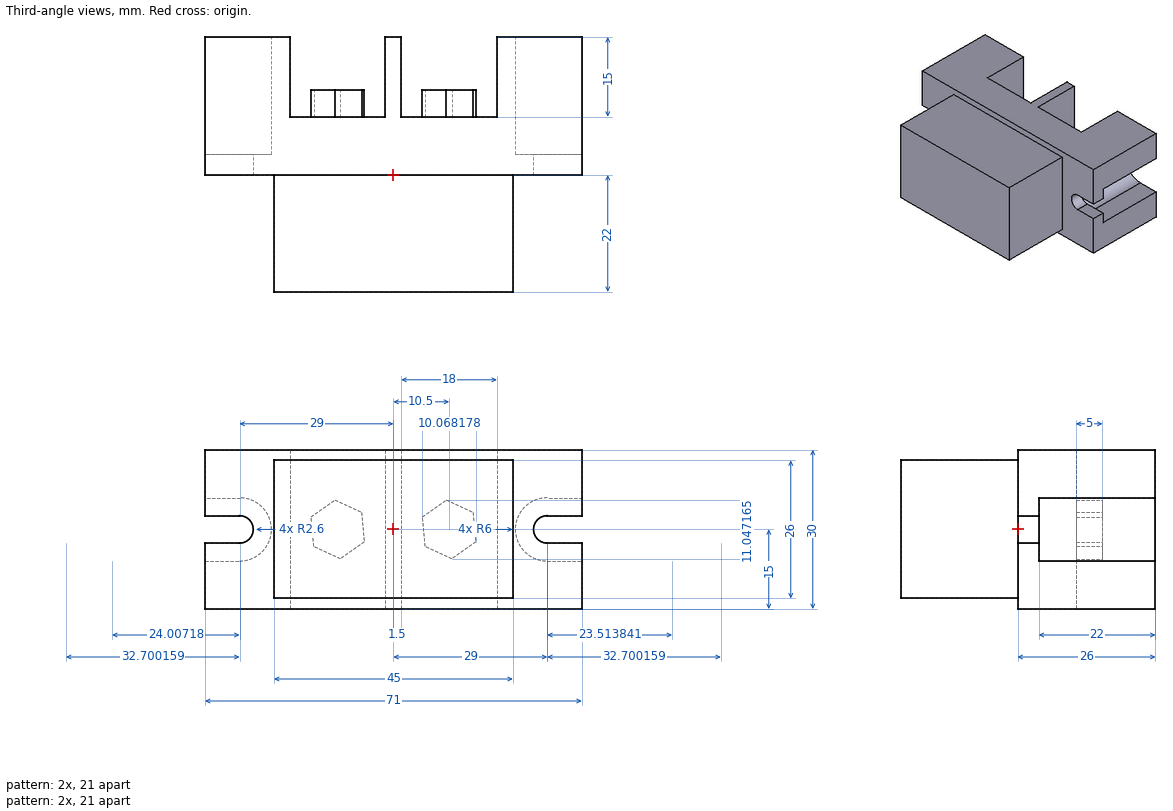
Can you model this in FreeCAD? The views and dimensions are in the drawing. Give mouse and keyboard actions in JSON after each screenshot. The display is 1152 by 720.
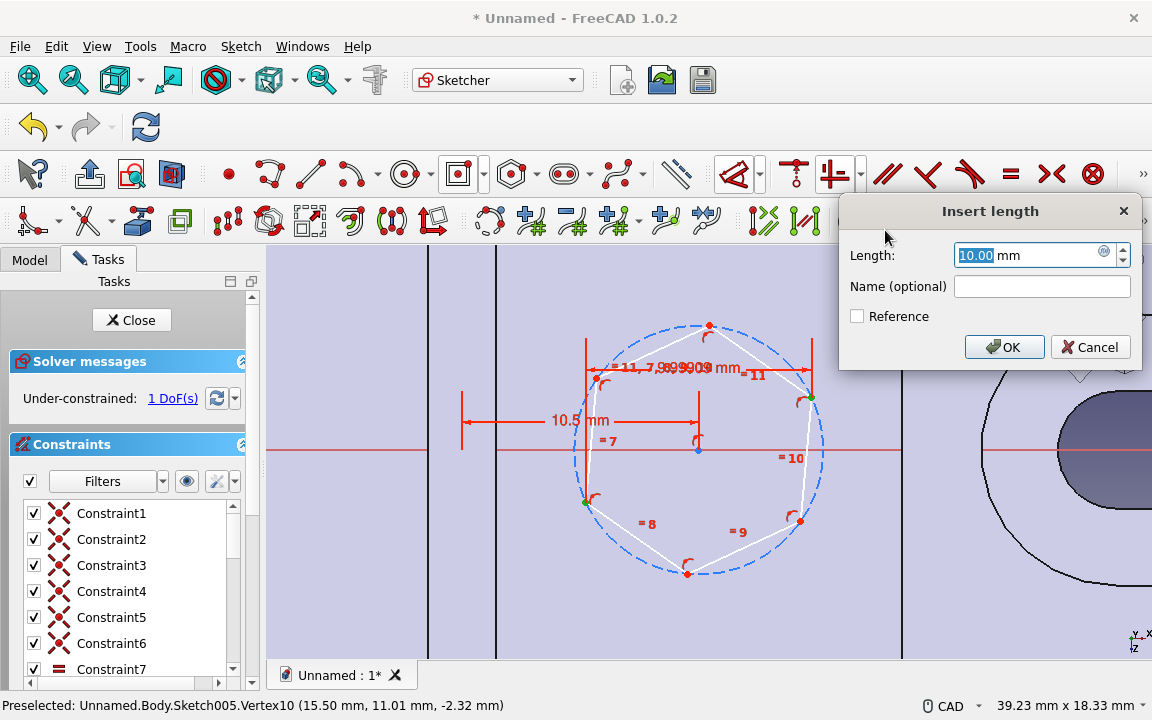
{"action": "type", "text": "10.068178"}
{"action": "key", "text": "Return"}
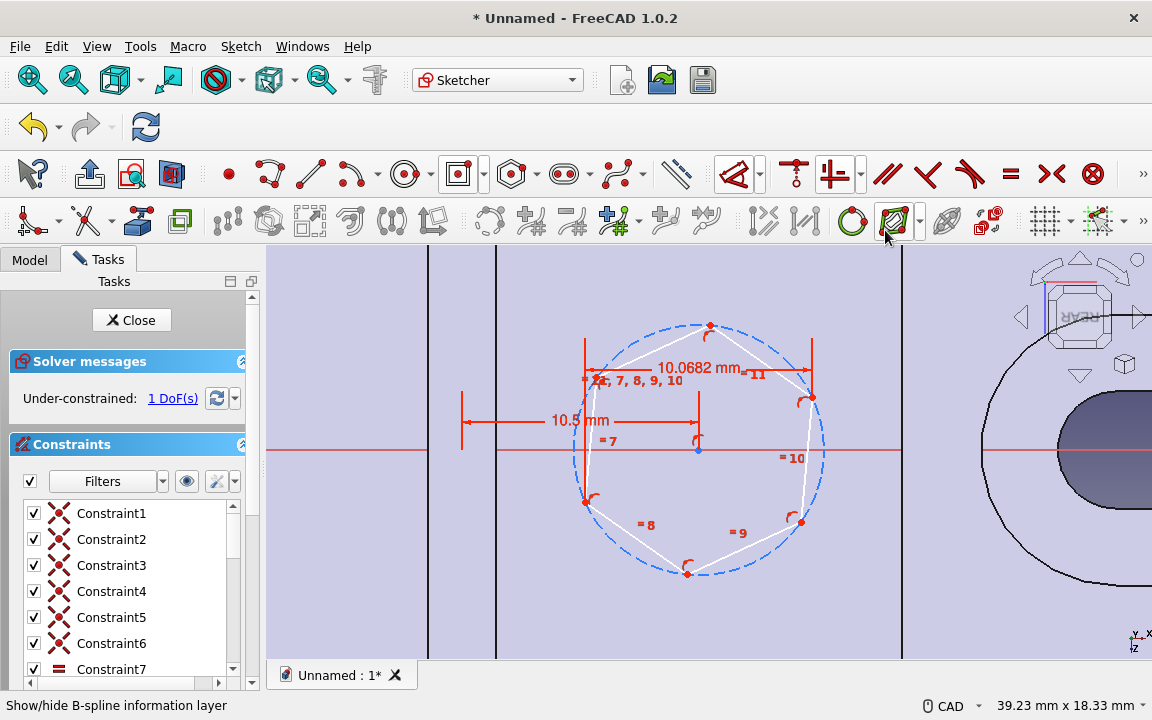
{"action": "left_click", "coordinate": [687, 575]}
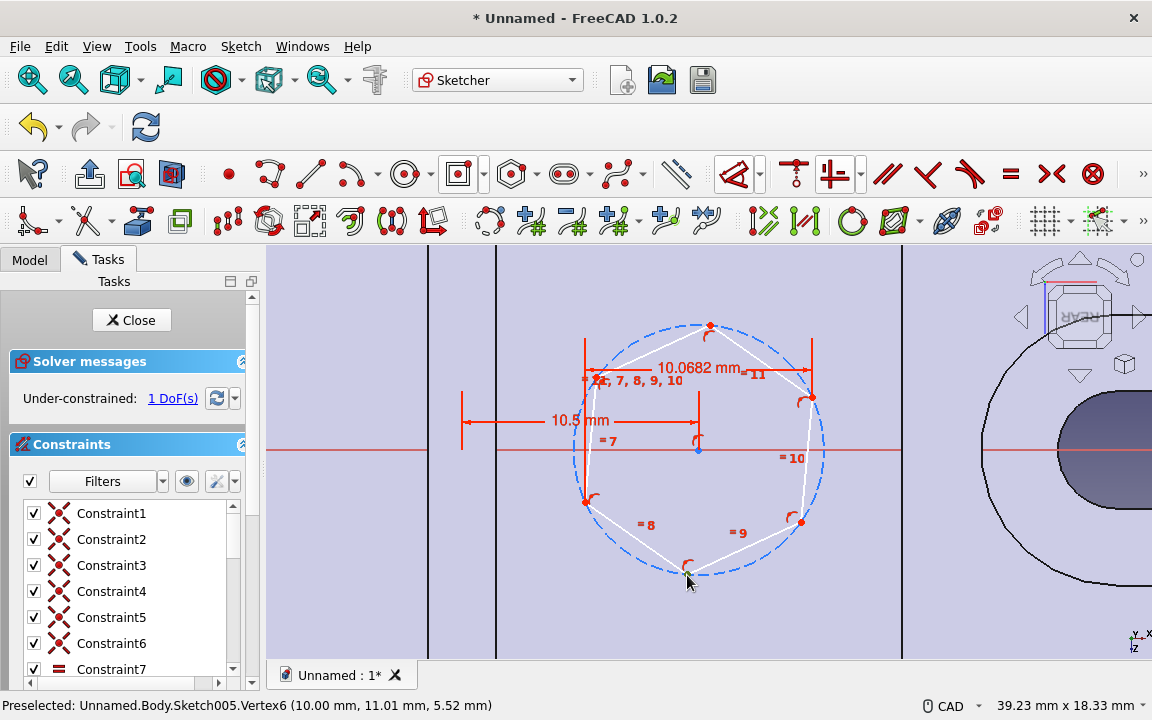
{"action": "left_click", "coordinate": [710, 325]}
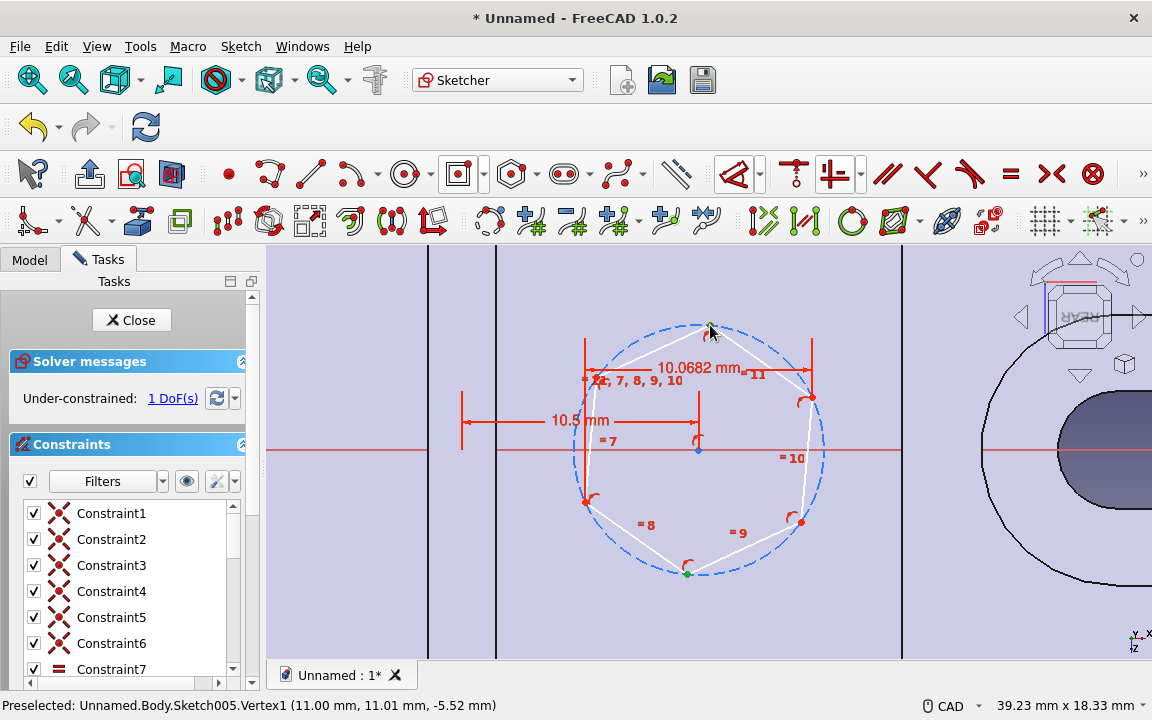
{"action": "key", "text": "i"}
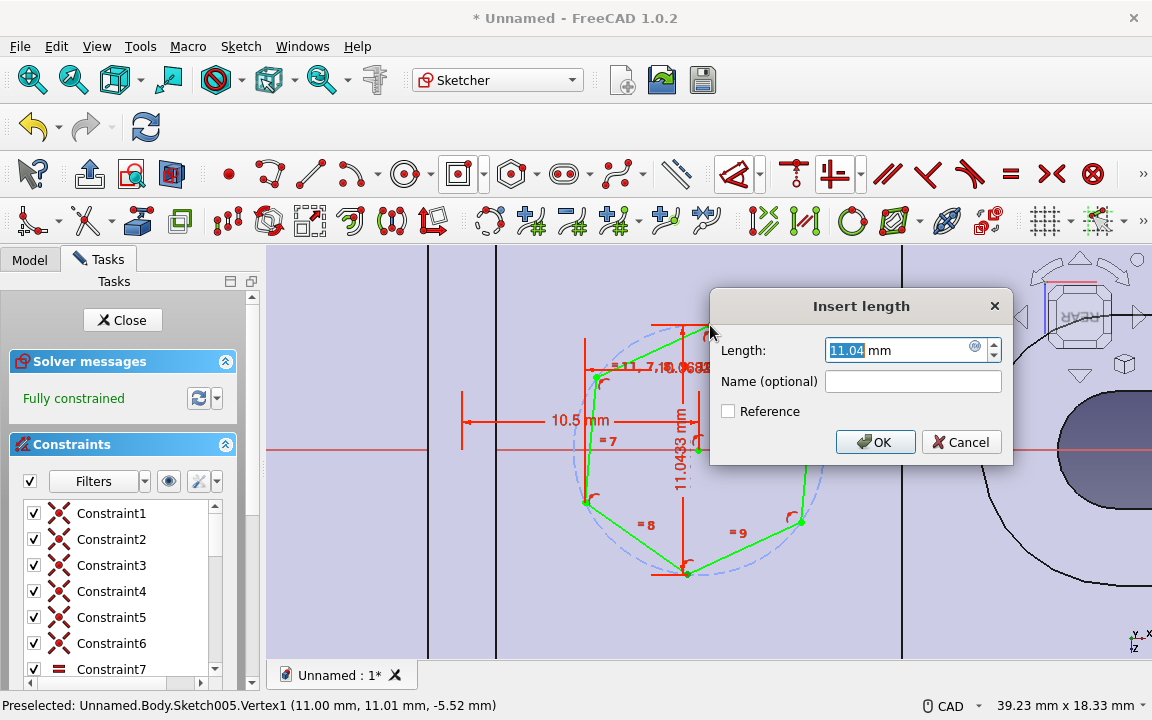
{"action": "type", "text": "11.047165"}
{"action": "key", "text": "Return"}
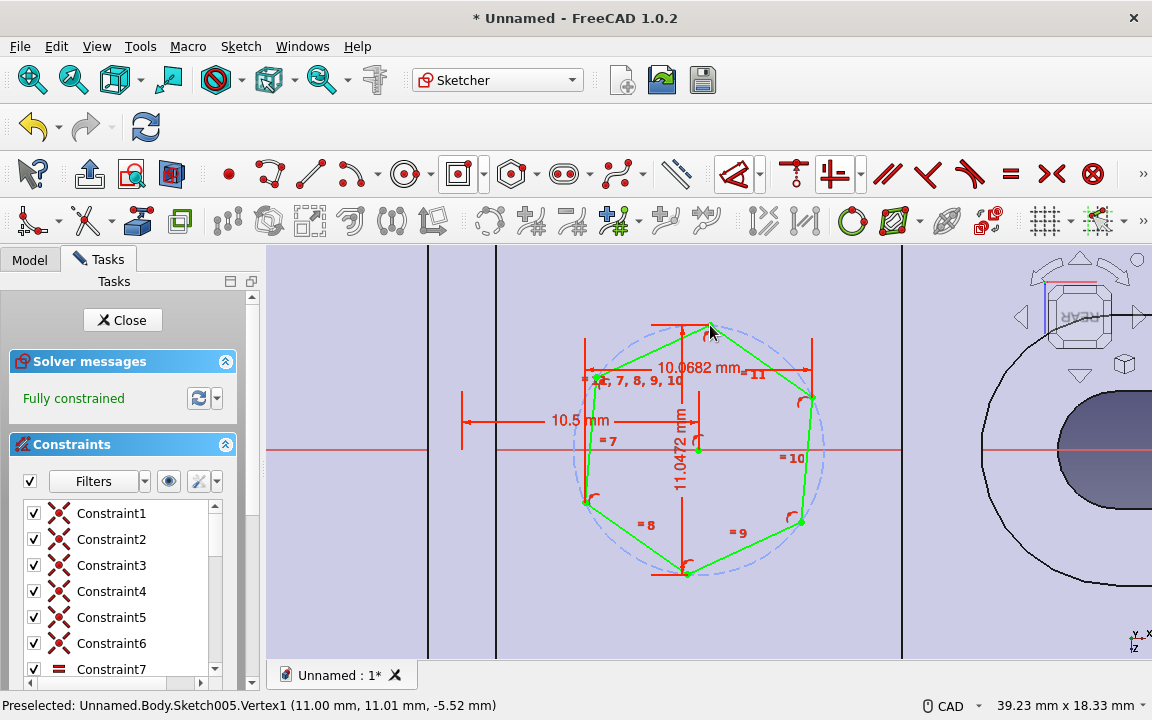
{"action": "left_click", "coordinate": [123, 320]}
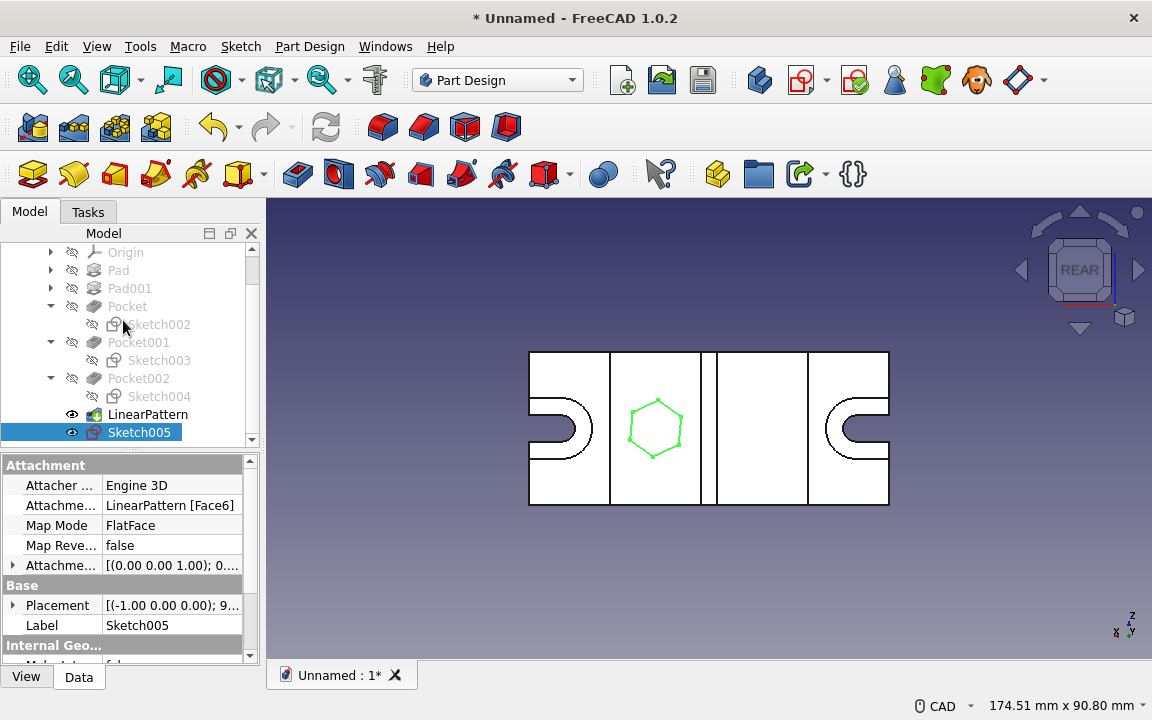
{"action": "left_click", "coordinate": [33, 174]}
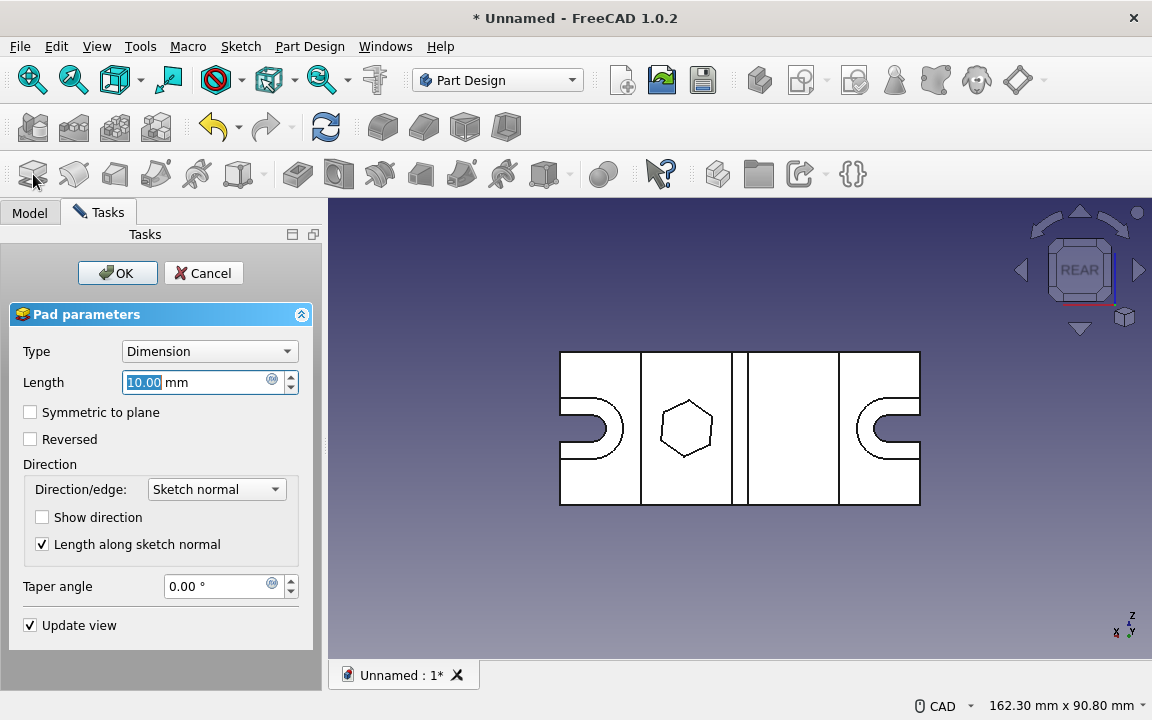
{"action": "type", "text": "5"}
{"action": "key", "text": "Tab"}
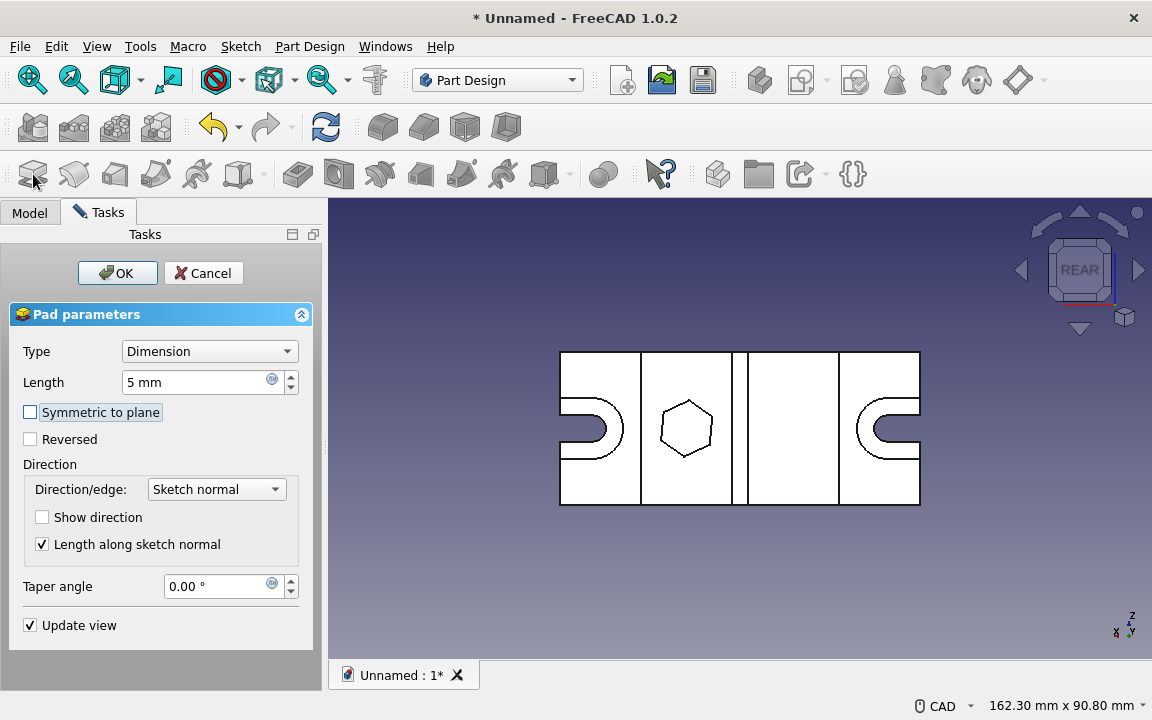
{"action": "left_click", "coordinate": [118, 273]}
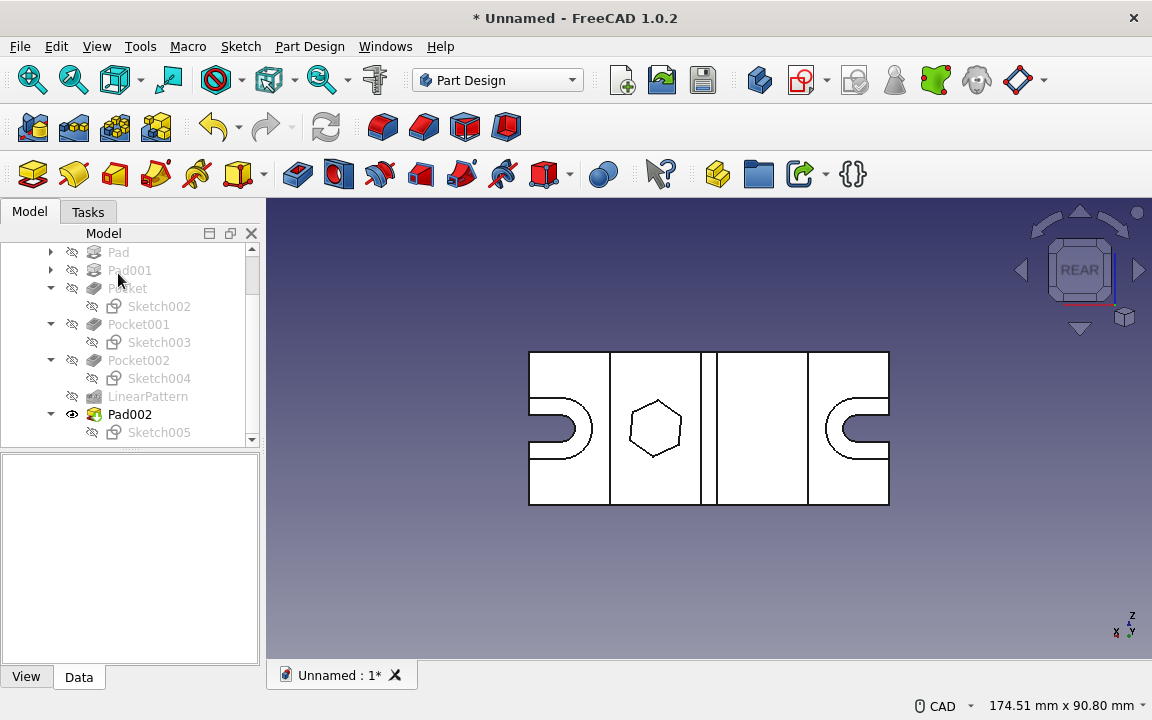
{"action": "key", "text": "v f"}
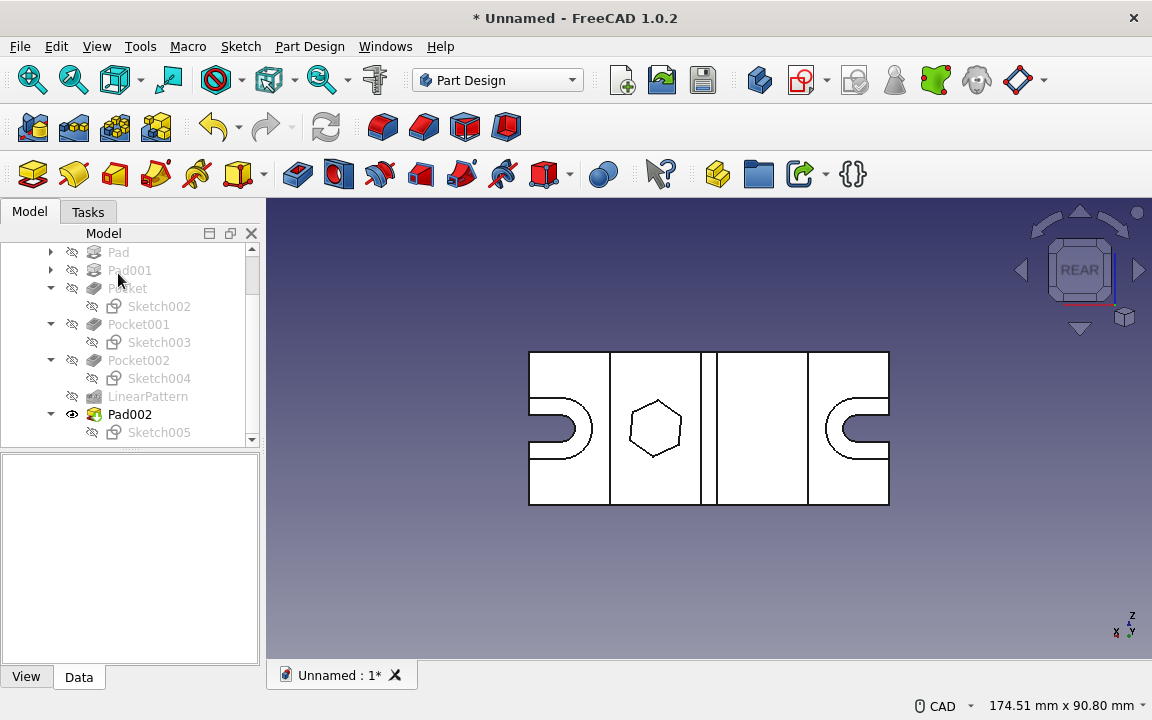
{"action": "left_click", "coordinate": [117, 414]}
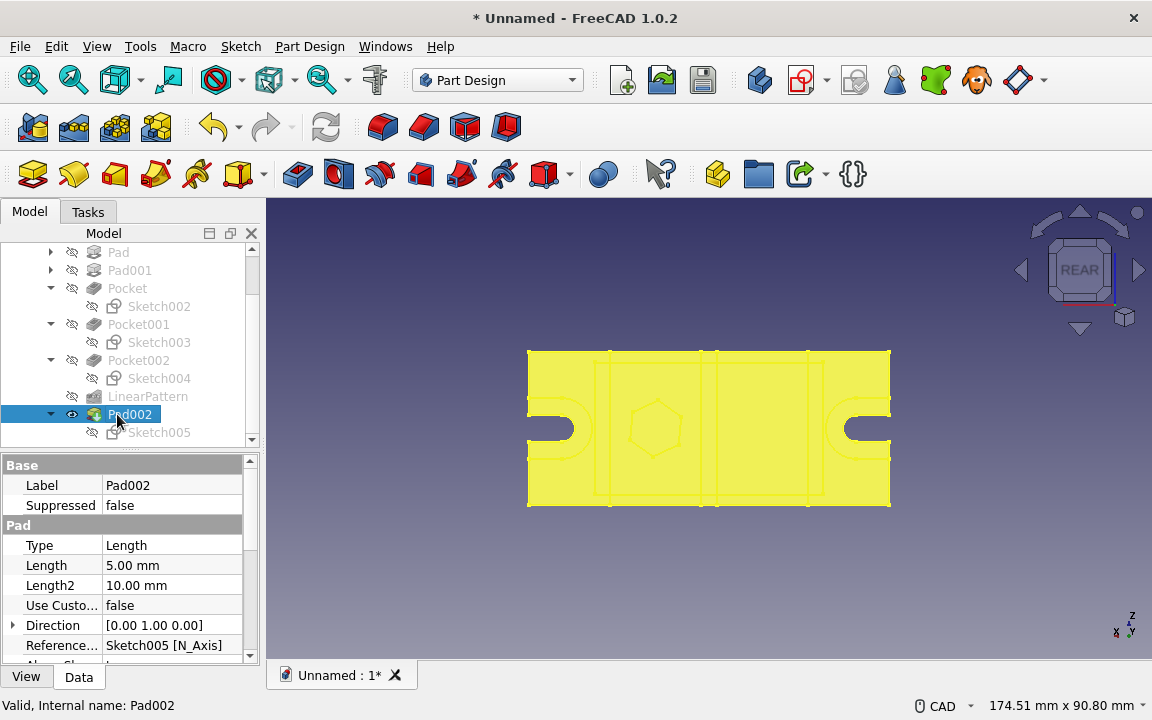
{"action": "left_click", "coordinate": [74, 128]}